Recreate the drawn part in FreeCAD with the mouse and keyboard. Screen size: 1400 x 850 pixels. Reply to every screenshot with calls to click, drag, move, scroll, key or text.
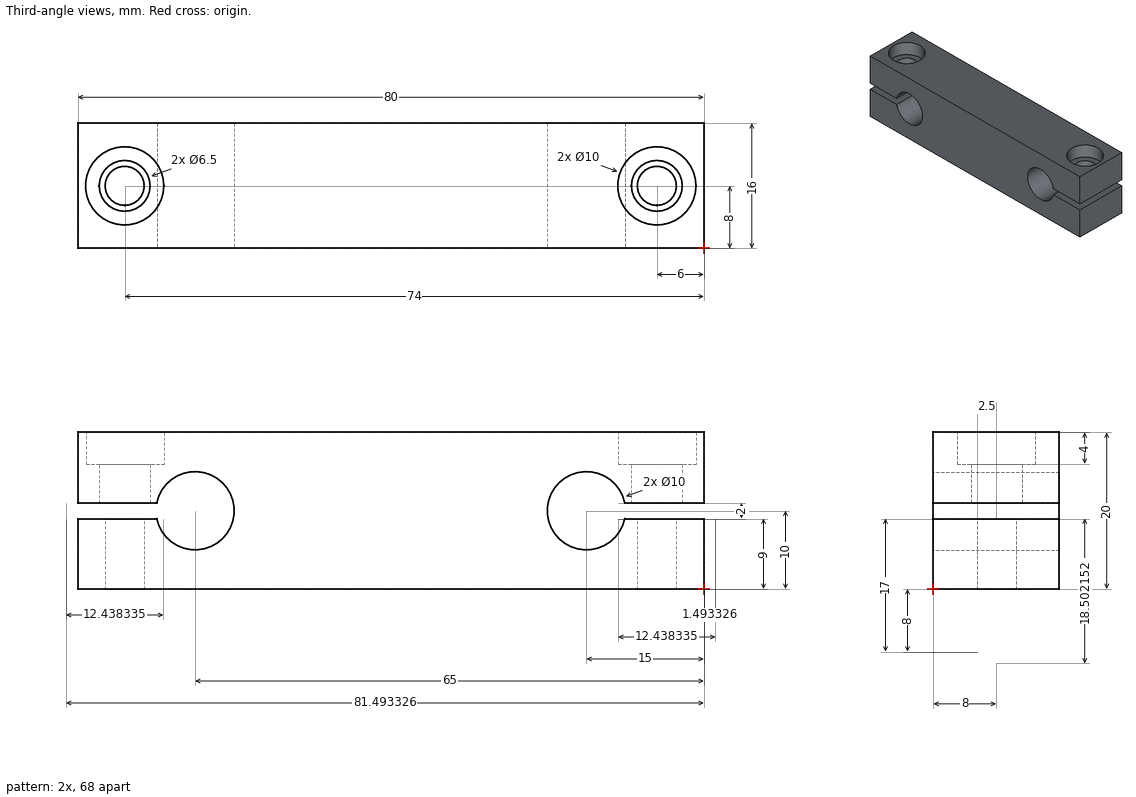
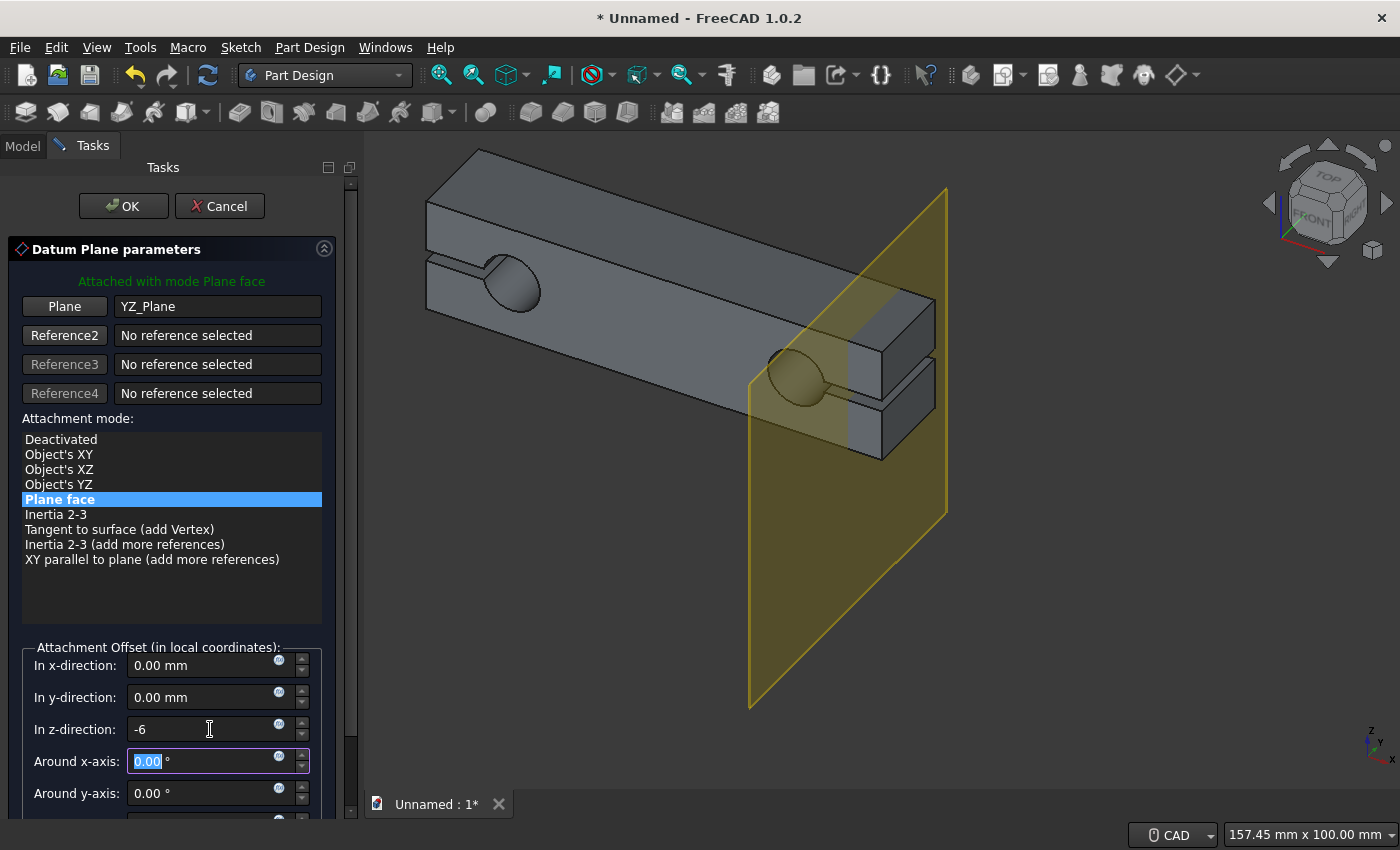
click(124, 206)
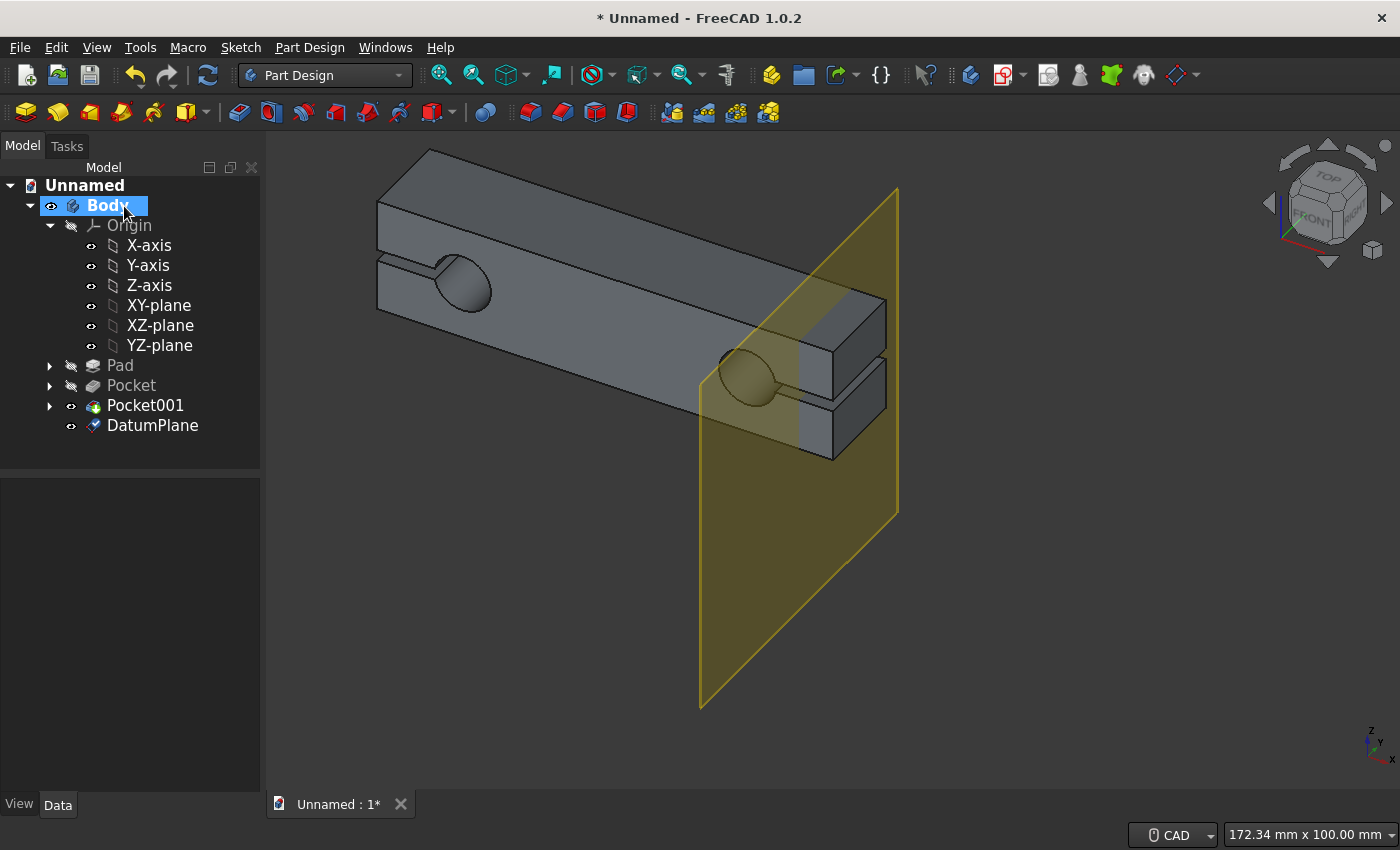
click(116, 426)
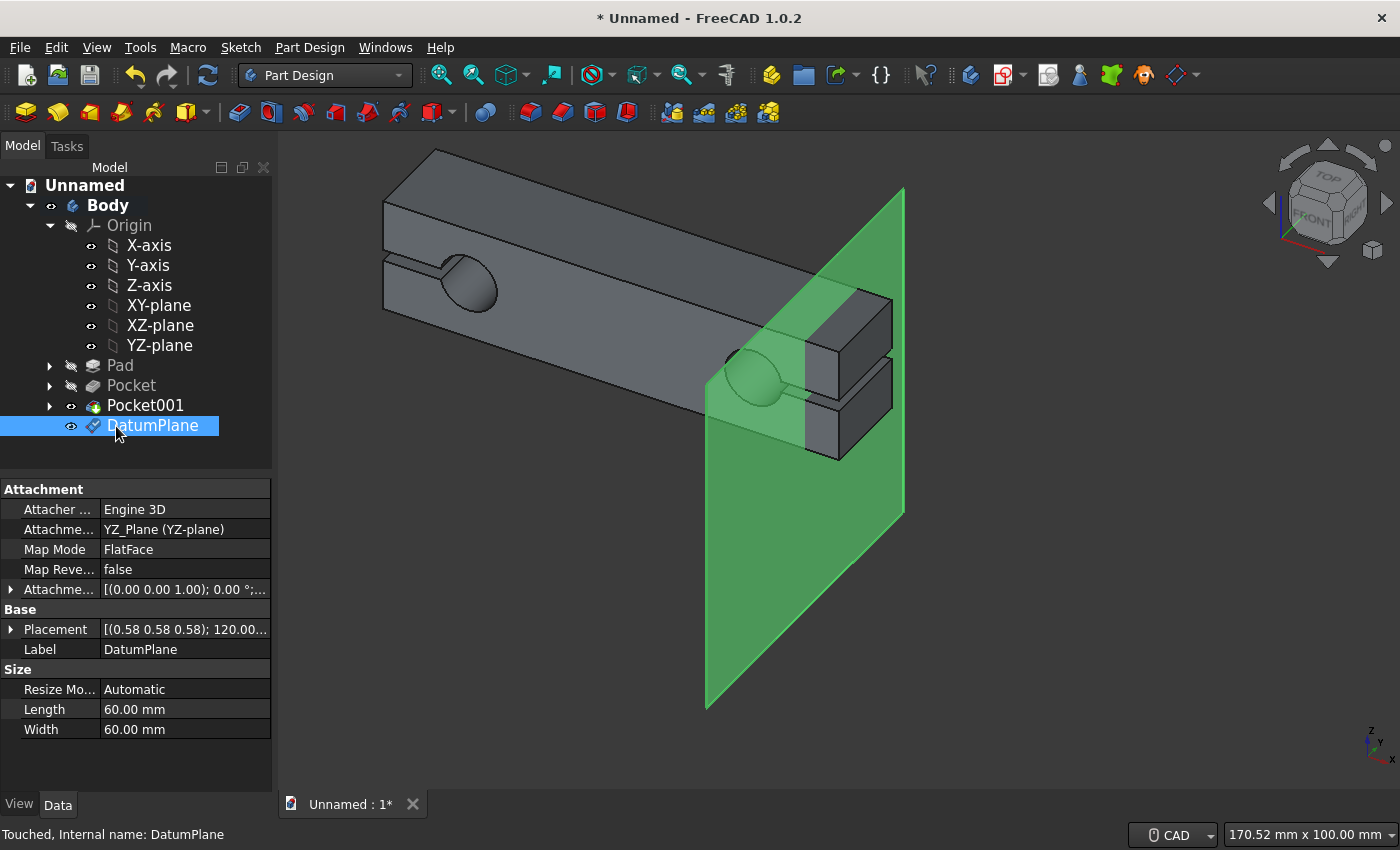
click(1004, 76)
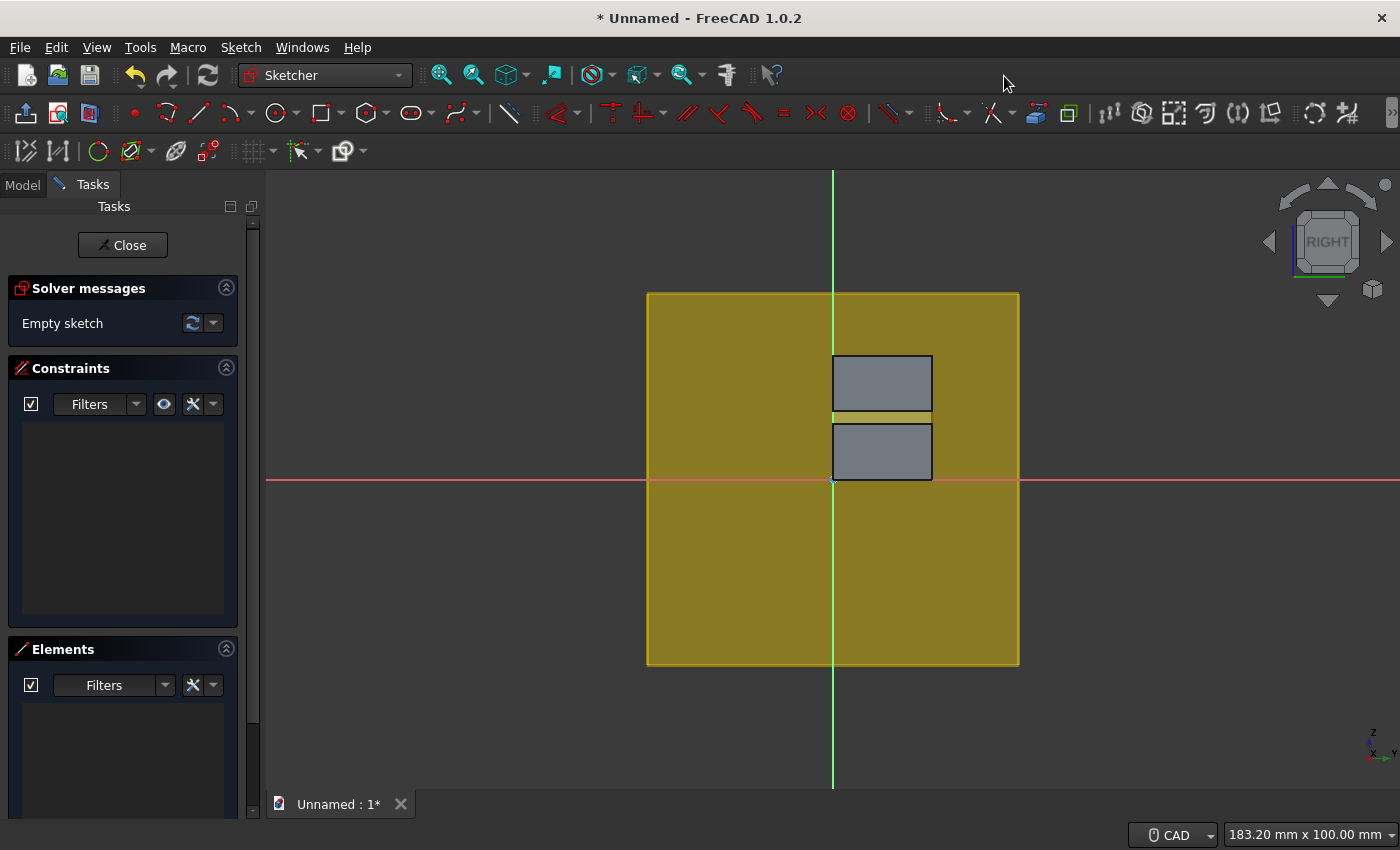
click(90, 114)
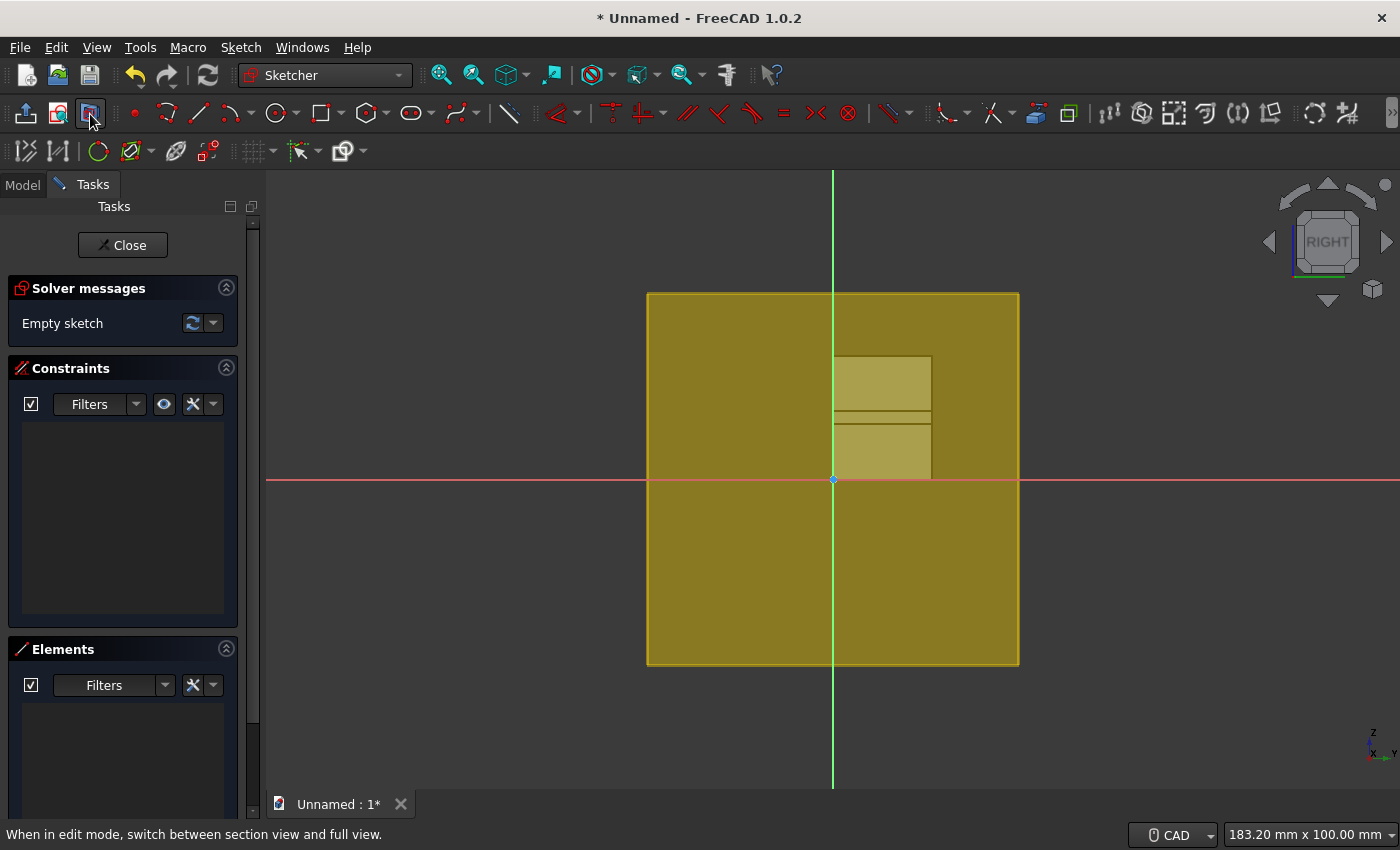
scroll(912, 518, up, 5)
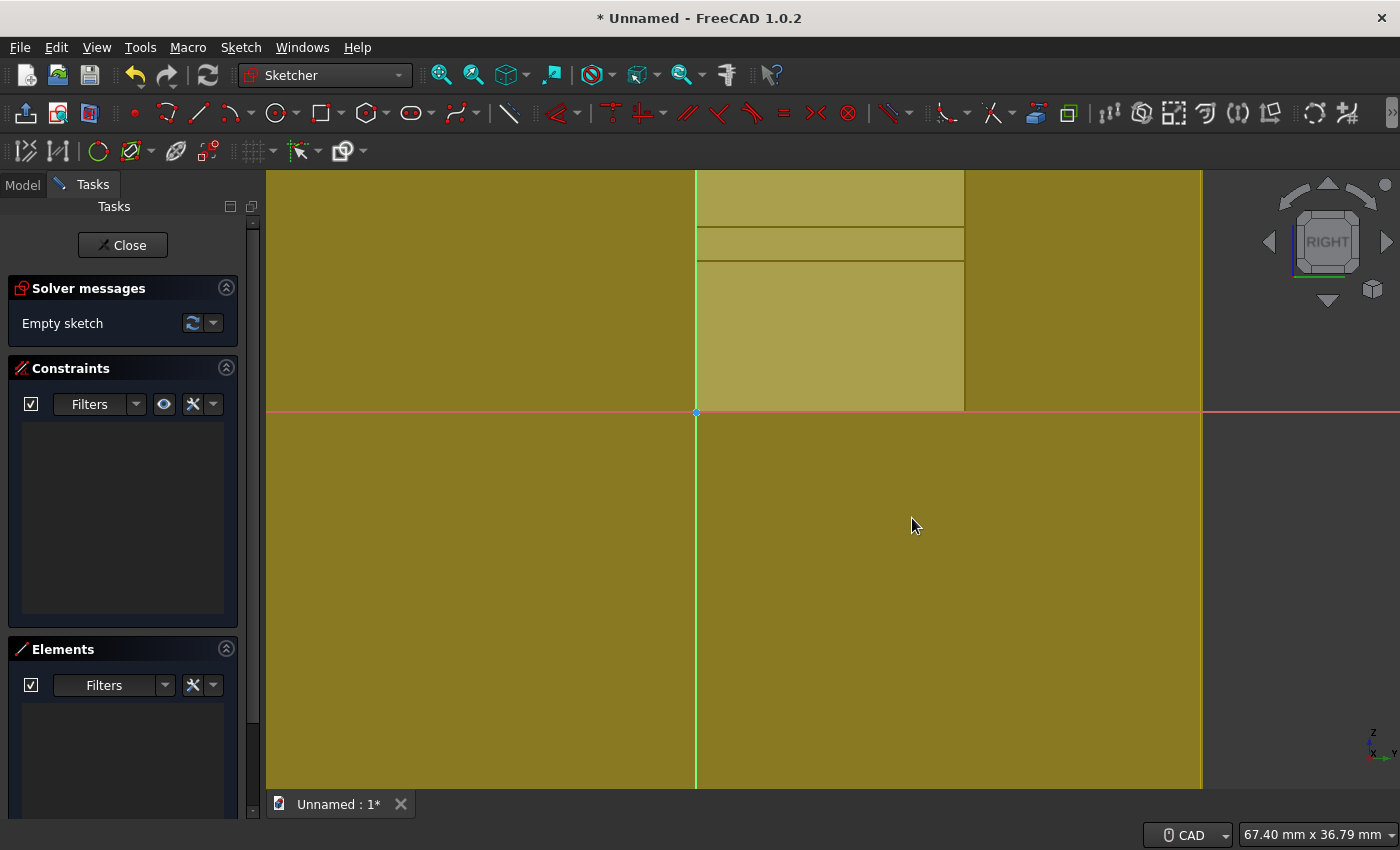
click(168, 114)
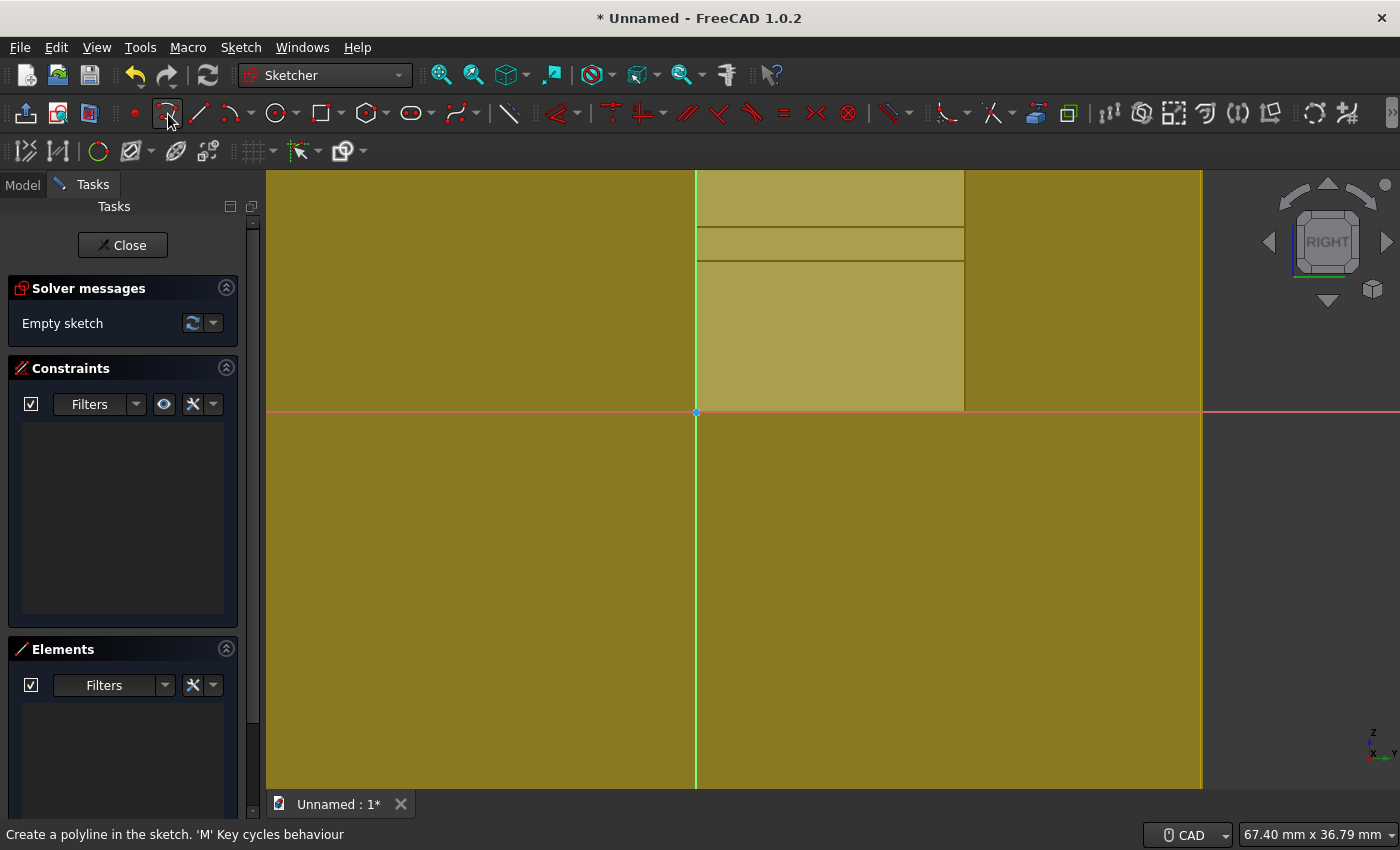
click(789, 547)
click(831, 572)
click(831, 261)
click(789, 261)
click(789, 548)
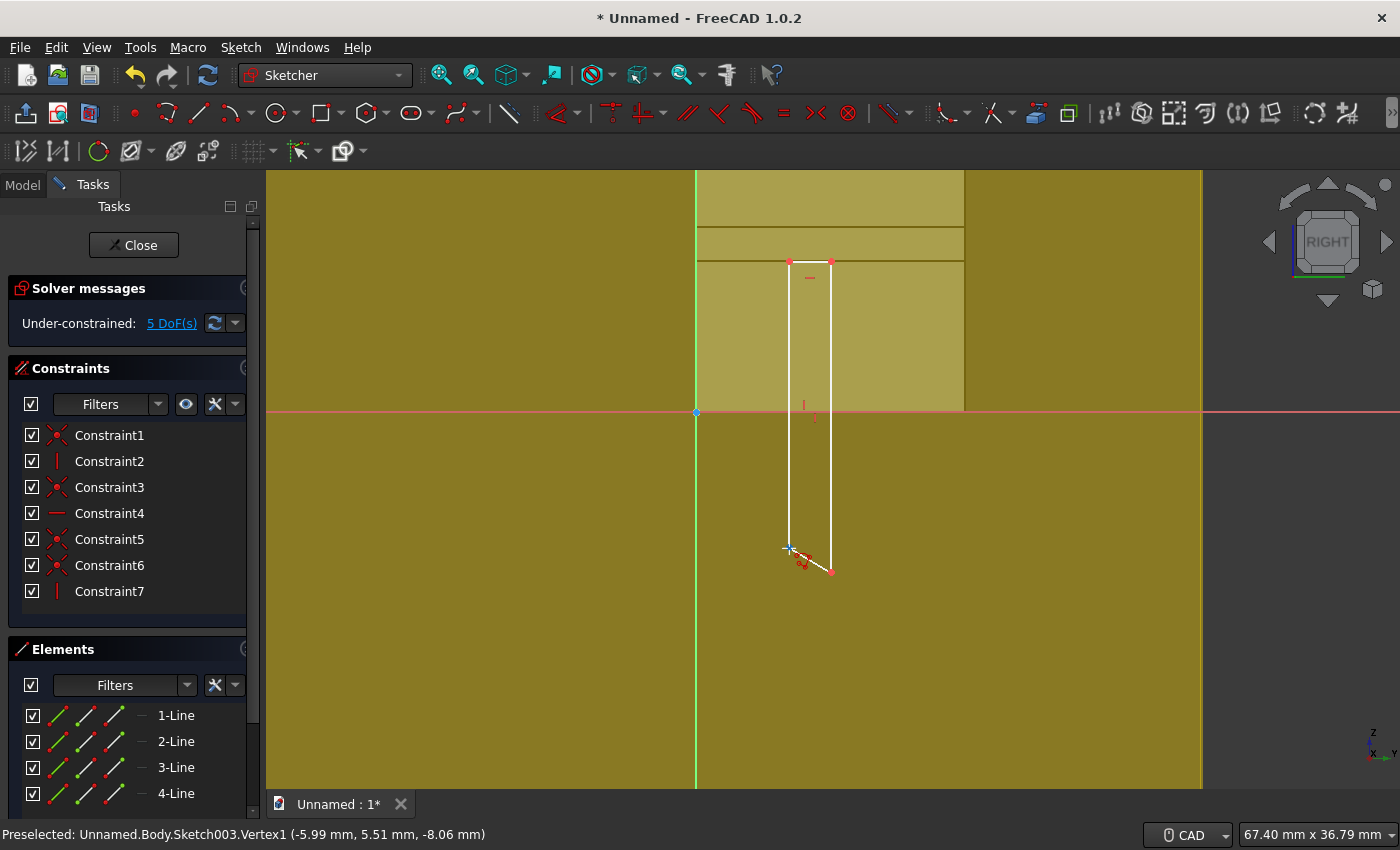
click(200, 114)